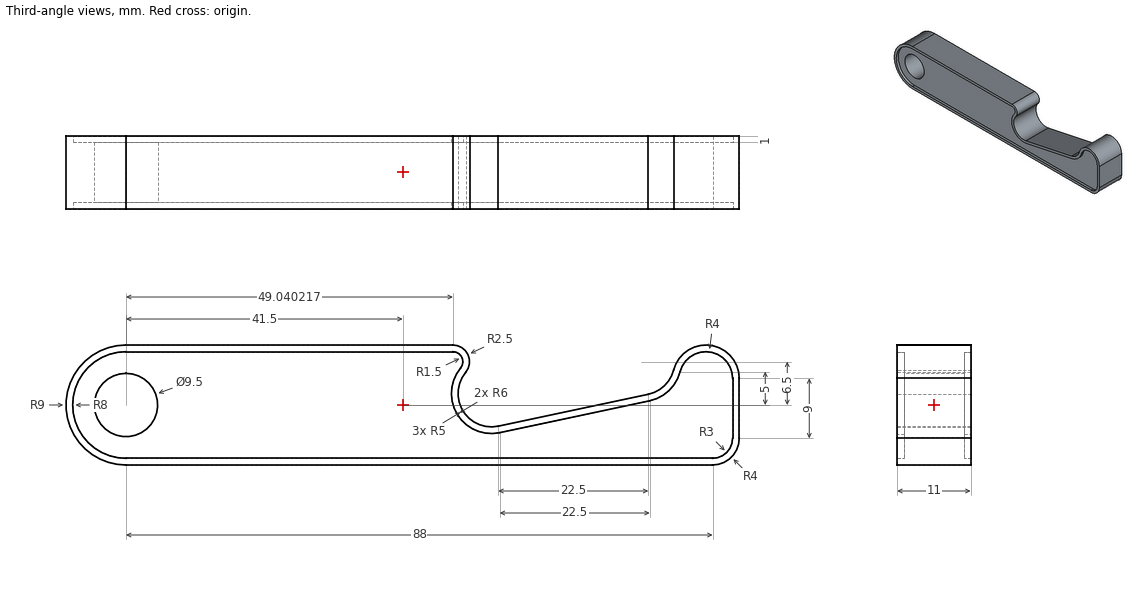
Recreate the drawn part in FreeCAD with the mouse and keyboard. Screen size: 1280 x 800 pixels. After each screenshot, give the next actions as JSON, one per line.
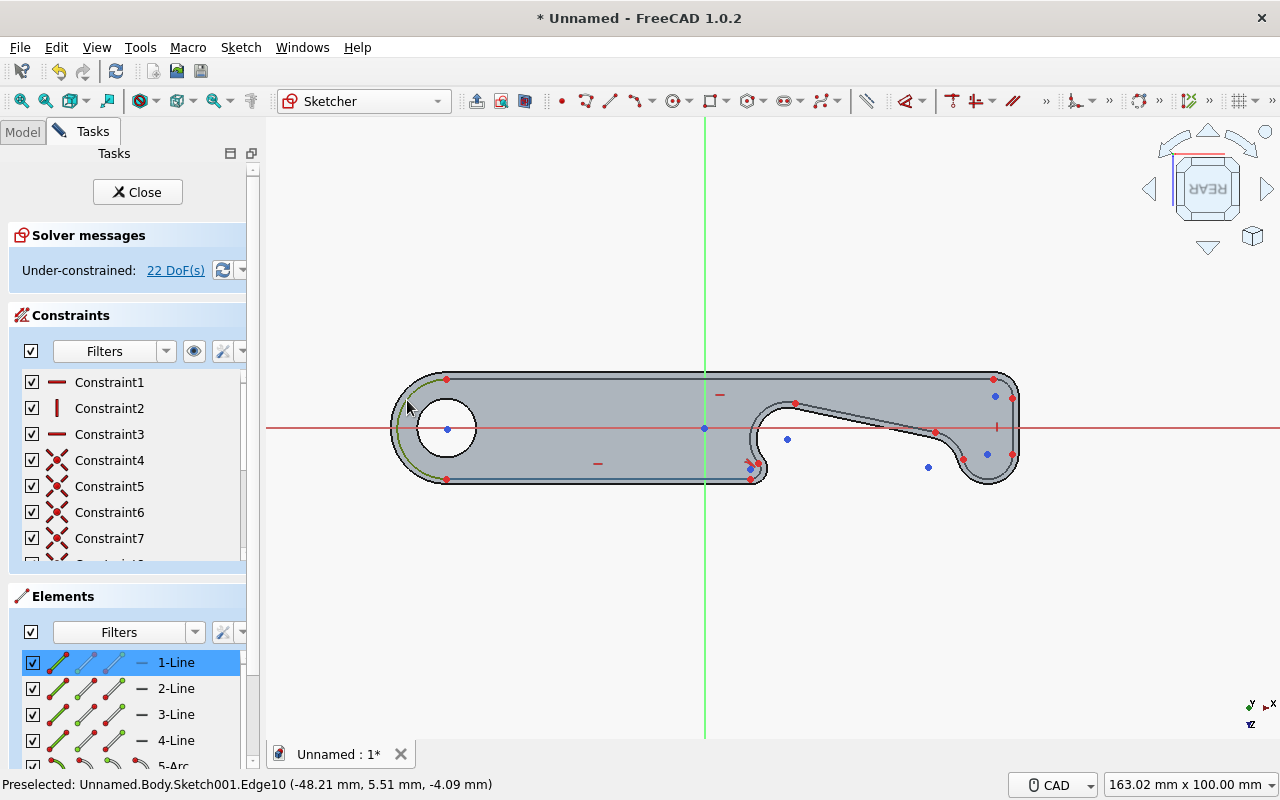
{"action": "key", "text": "t"}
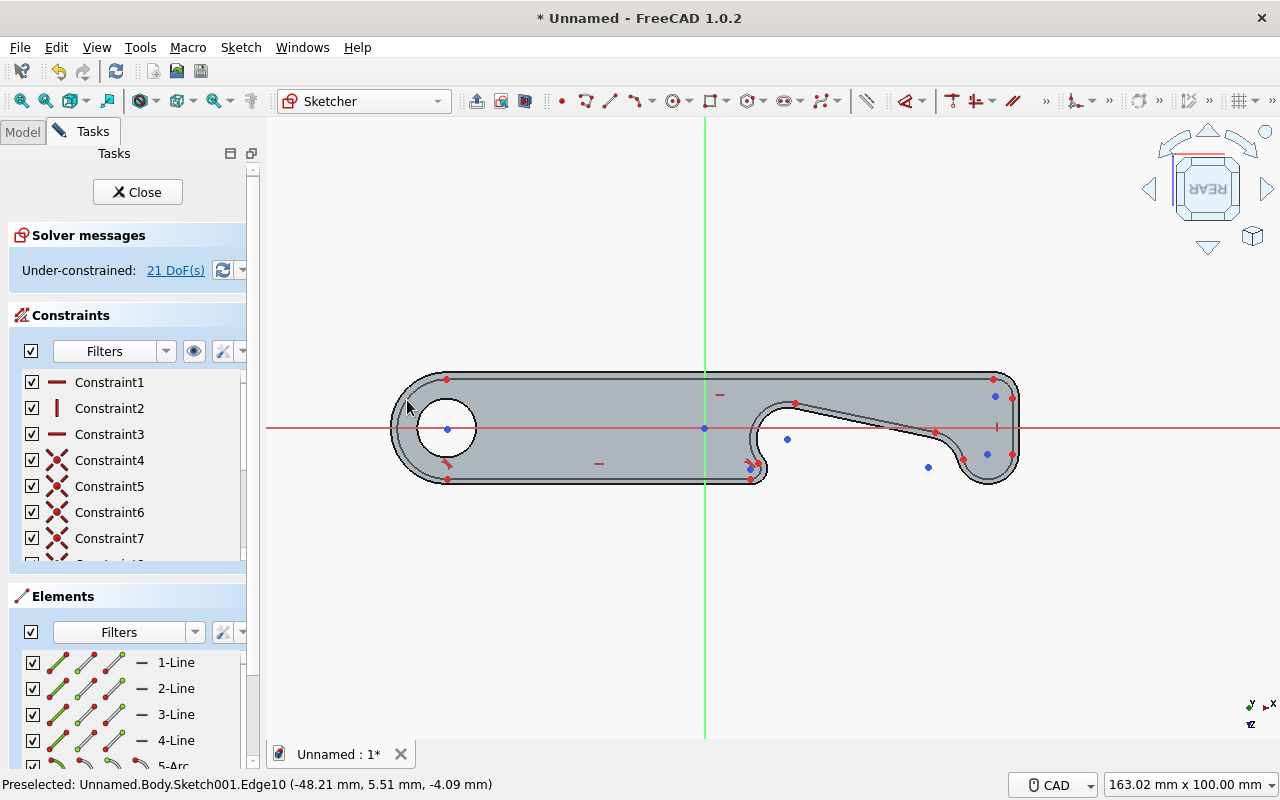
{"action": "left_click", "coordinate": [838, 412]}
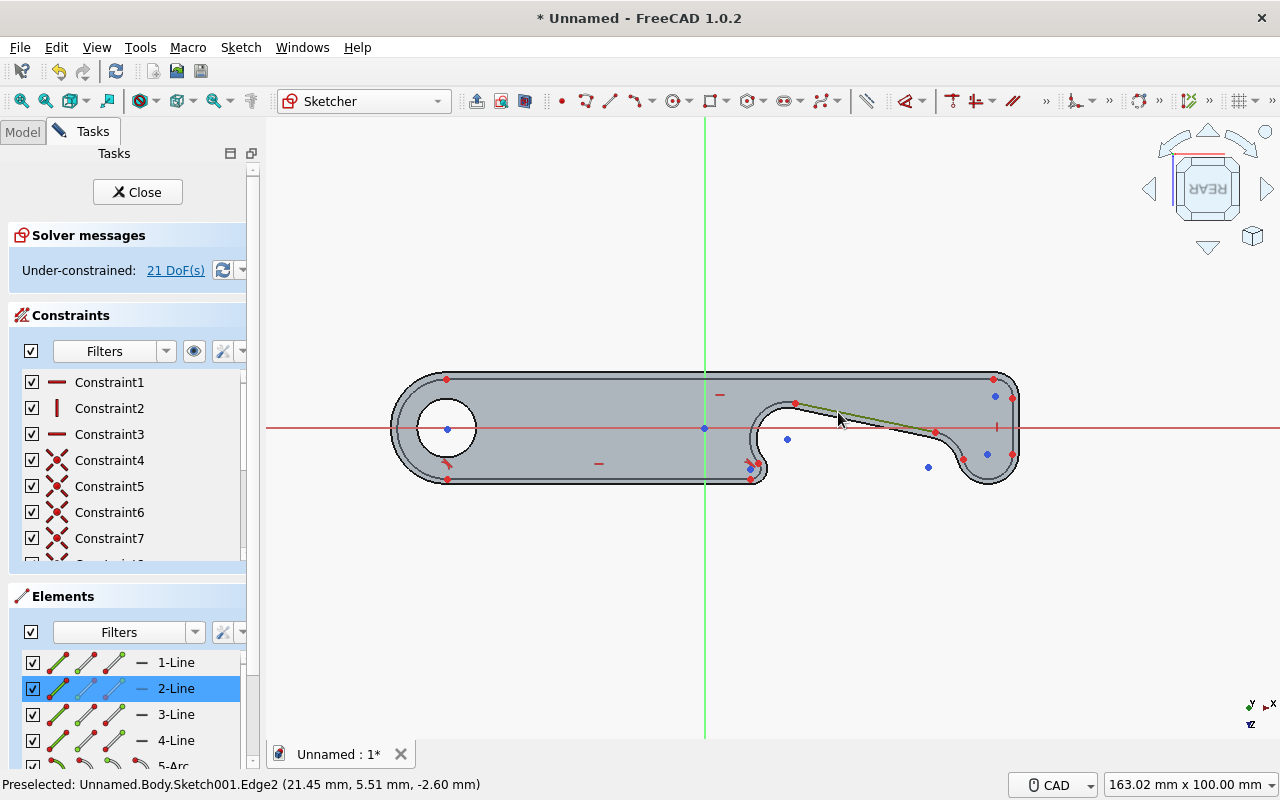
{"action": "left_click", "coordinate": [769, 407]}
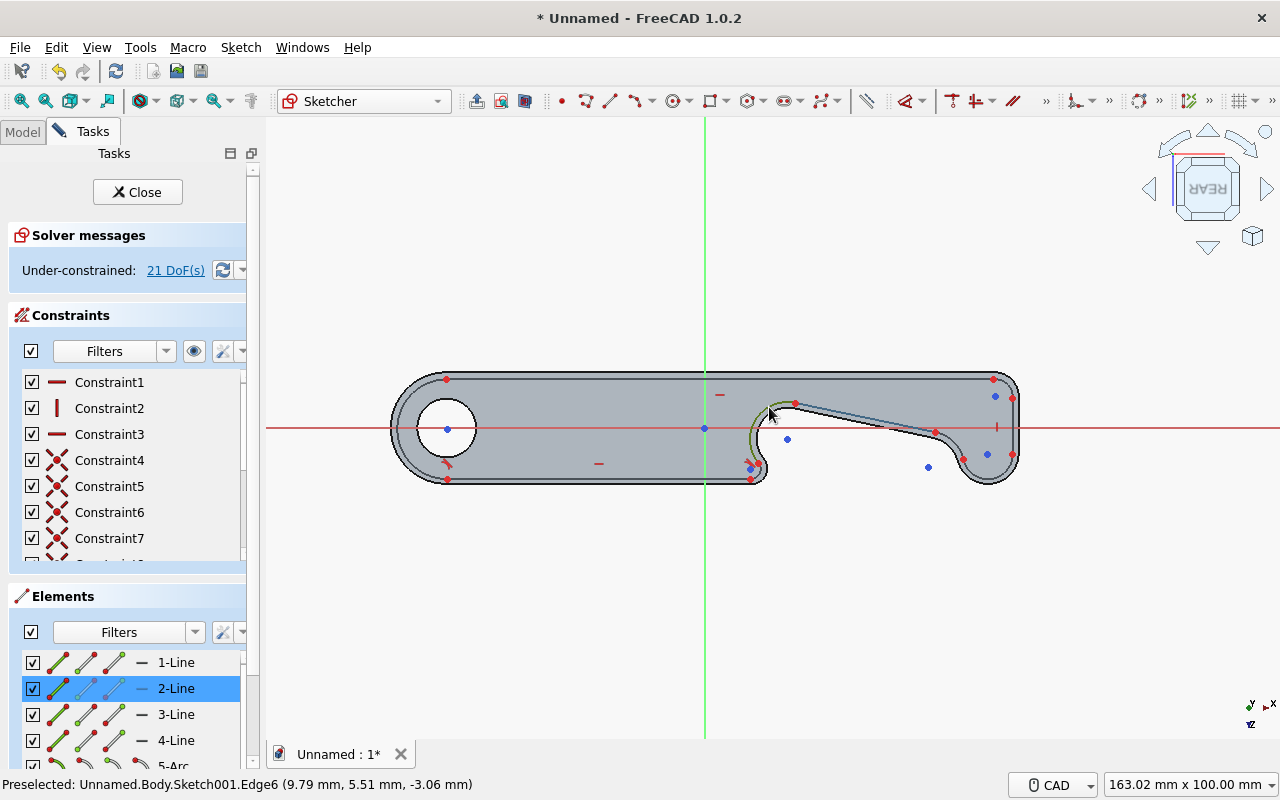
{"action": "key", "text": "t"}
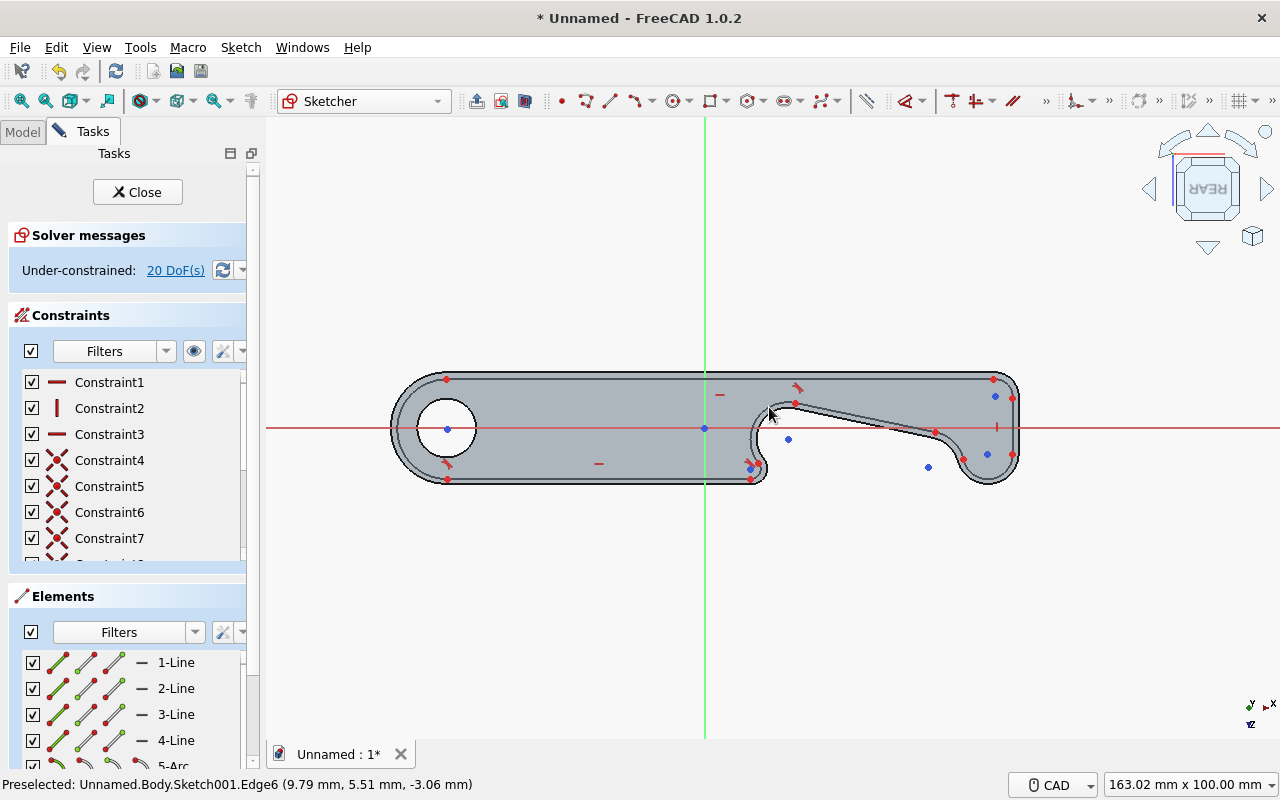
{"action": "left_click", "coordinate": [838, 412]}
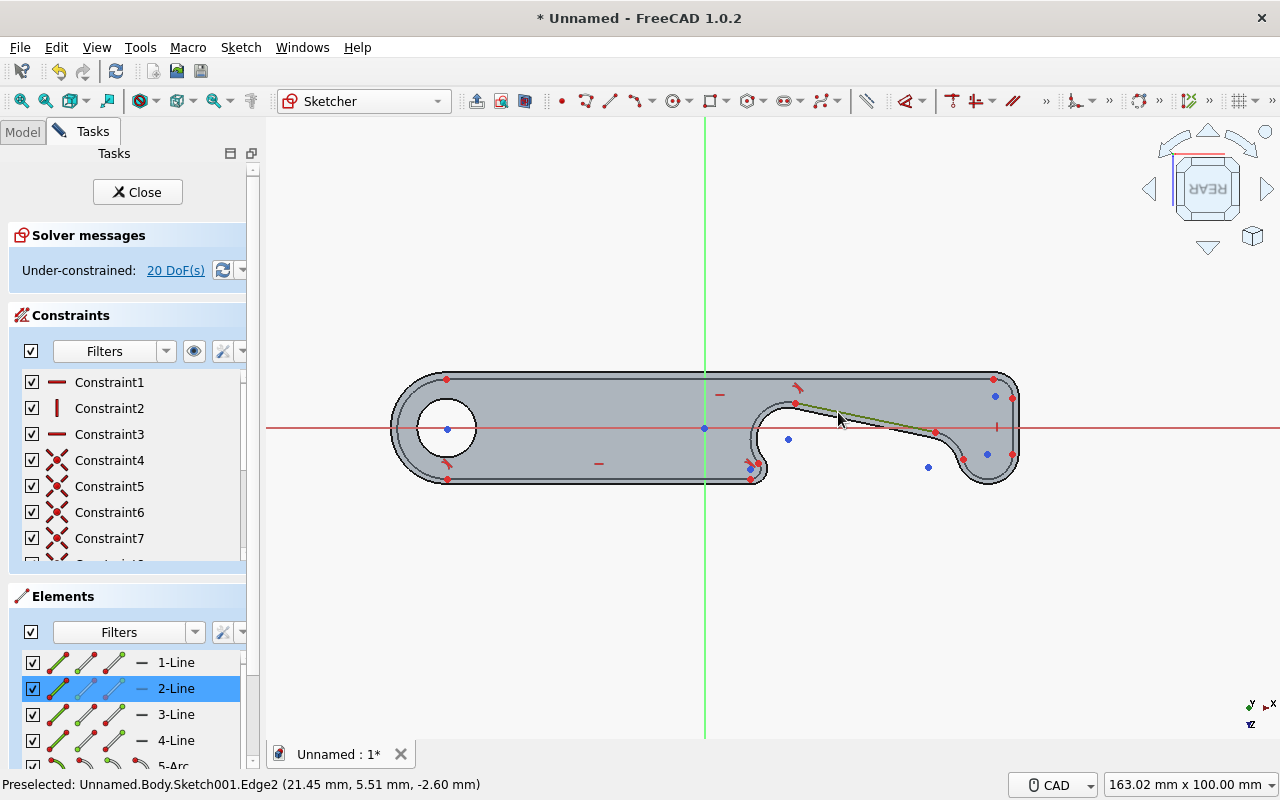
{"action": "left_click", "coordinate": [959, 448]}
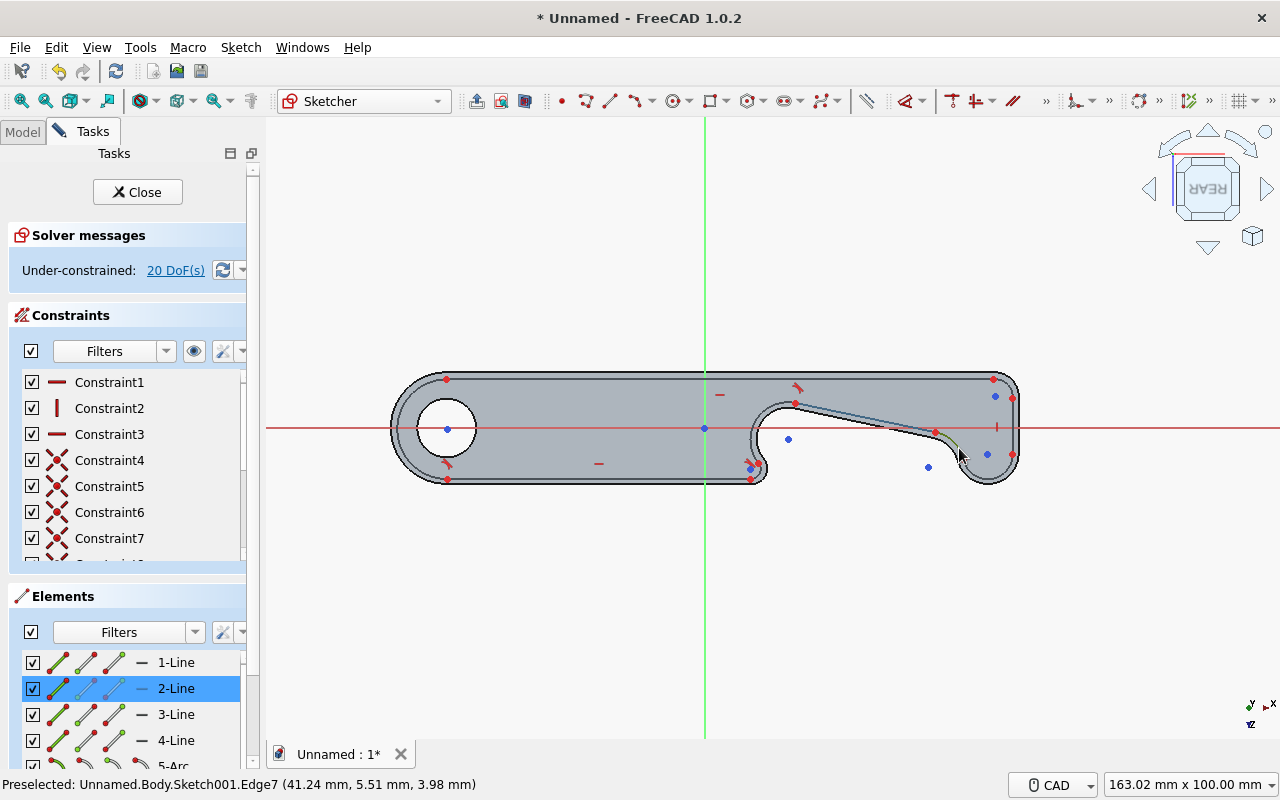
{"action": "key", "text": "t"}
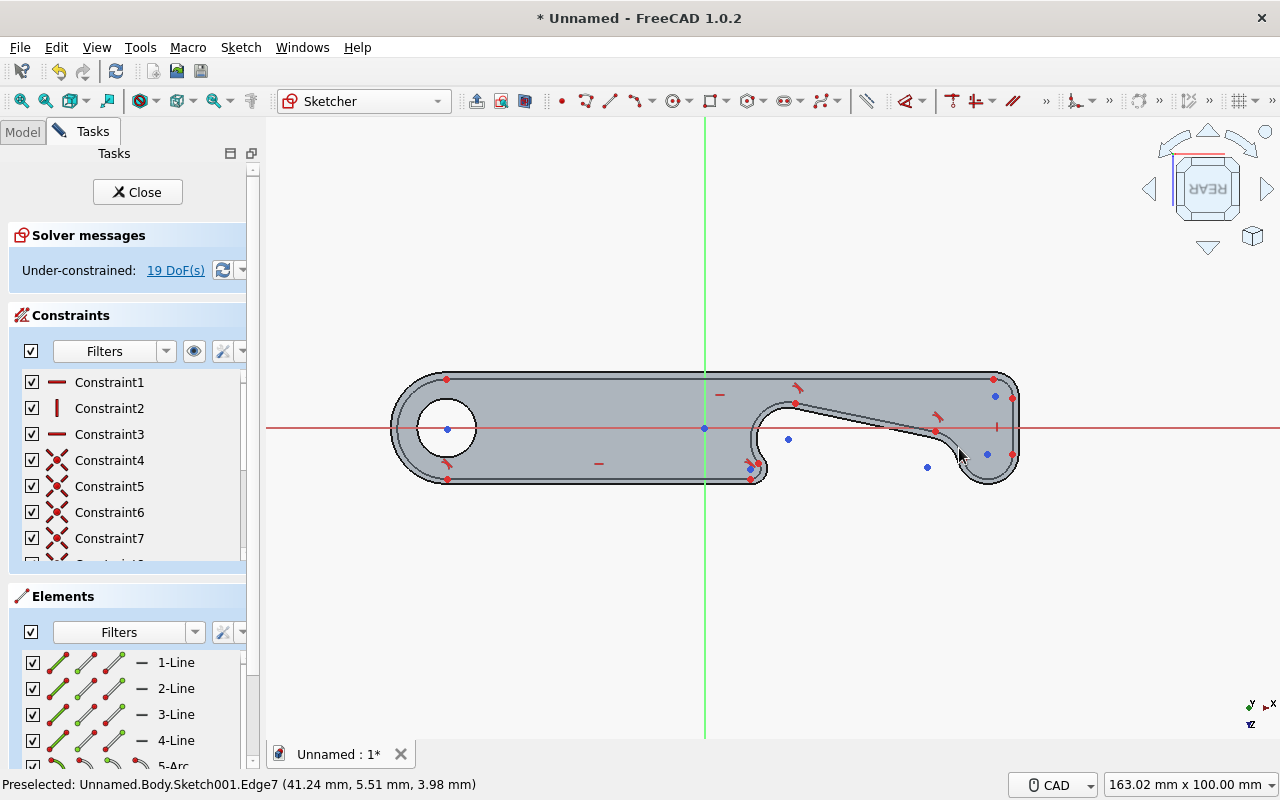
{"action": "scroll", "coordinate": [1013, 438], "scroll_direction": "up", "scroll_amount": 2}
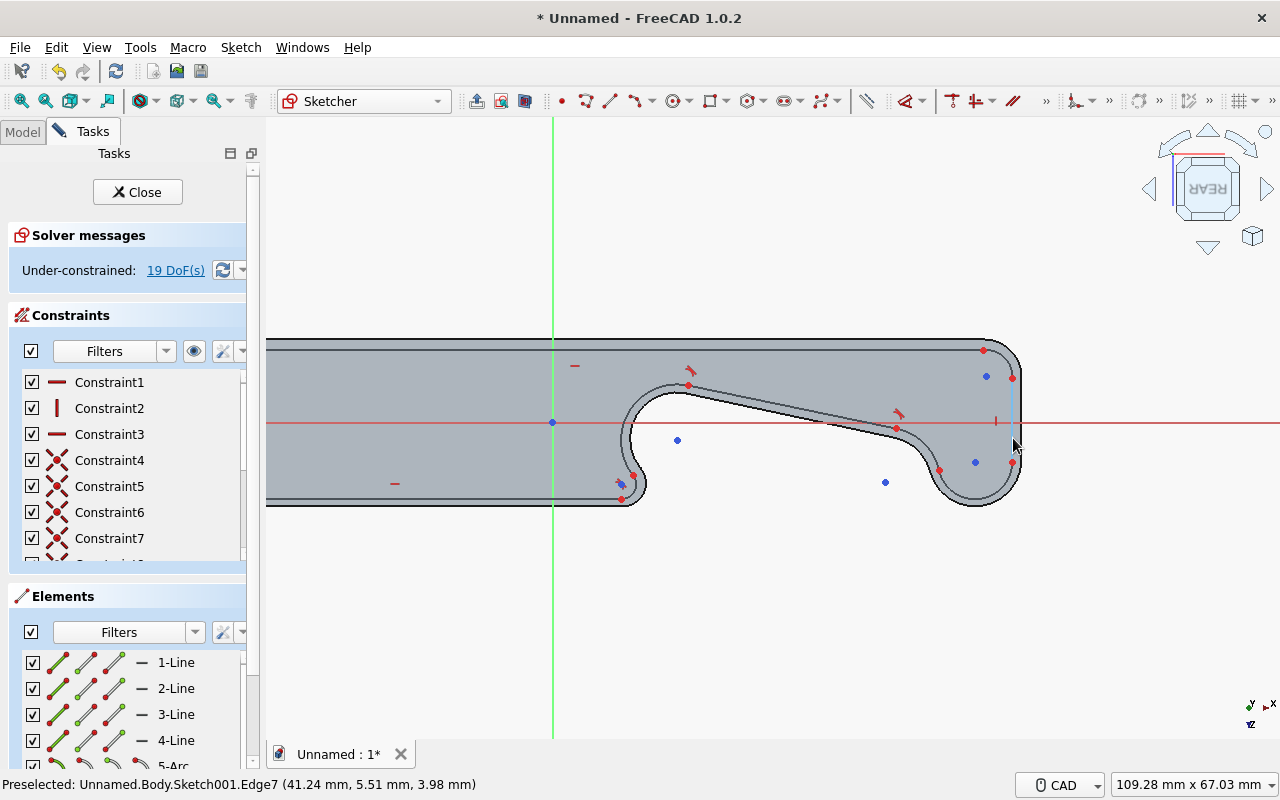
{"action": "left_click", "coordinate": [1012, 437]}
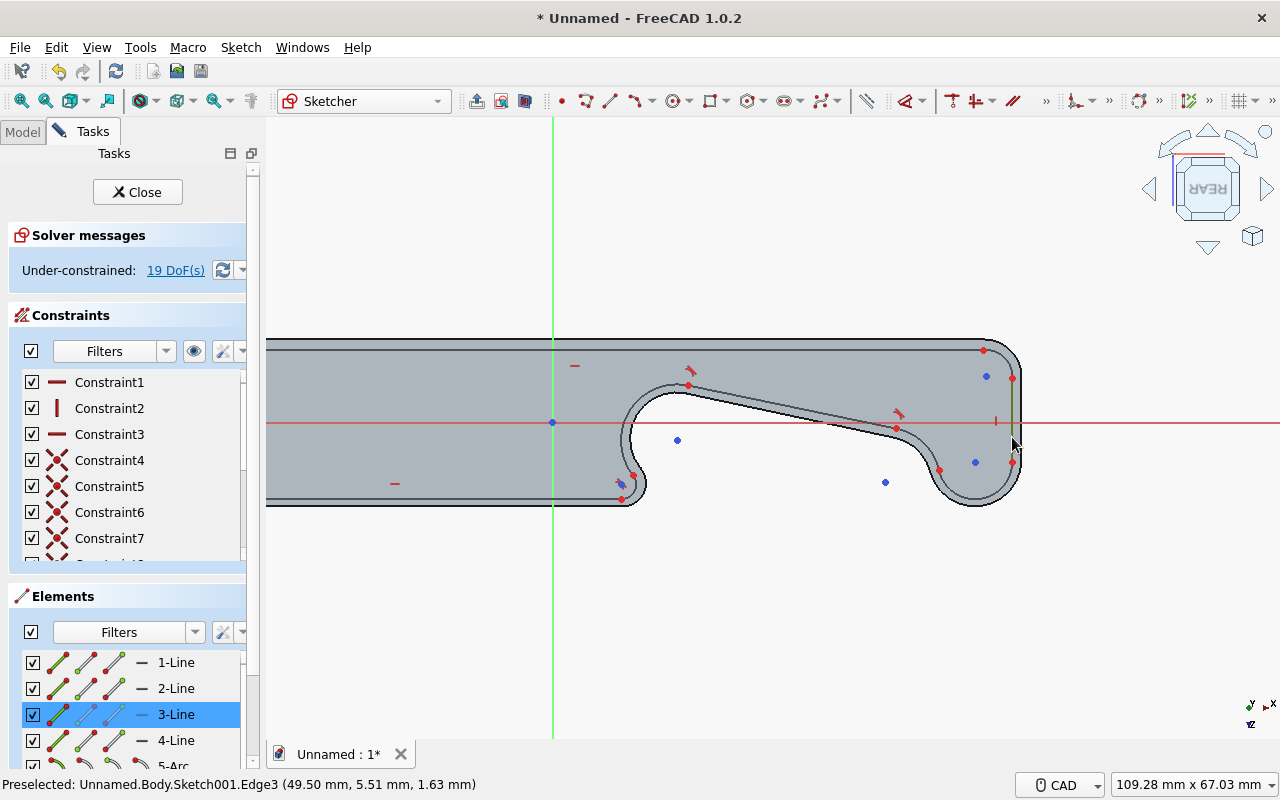
{"action": "left_click", "coordinate": [958, 495]}